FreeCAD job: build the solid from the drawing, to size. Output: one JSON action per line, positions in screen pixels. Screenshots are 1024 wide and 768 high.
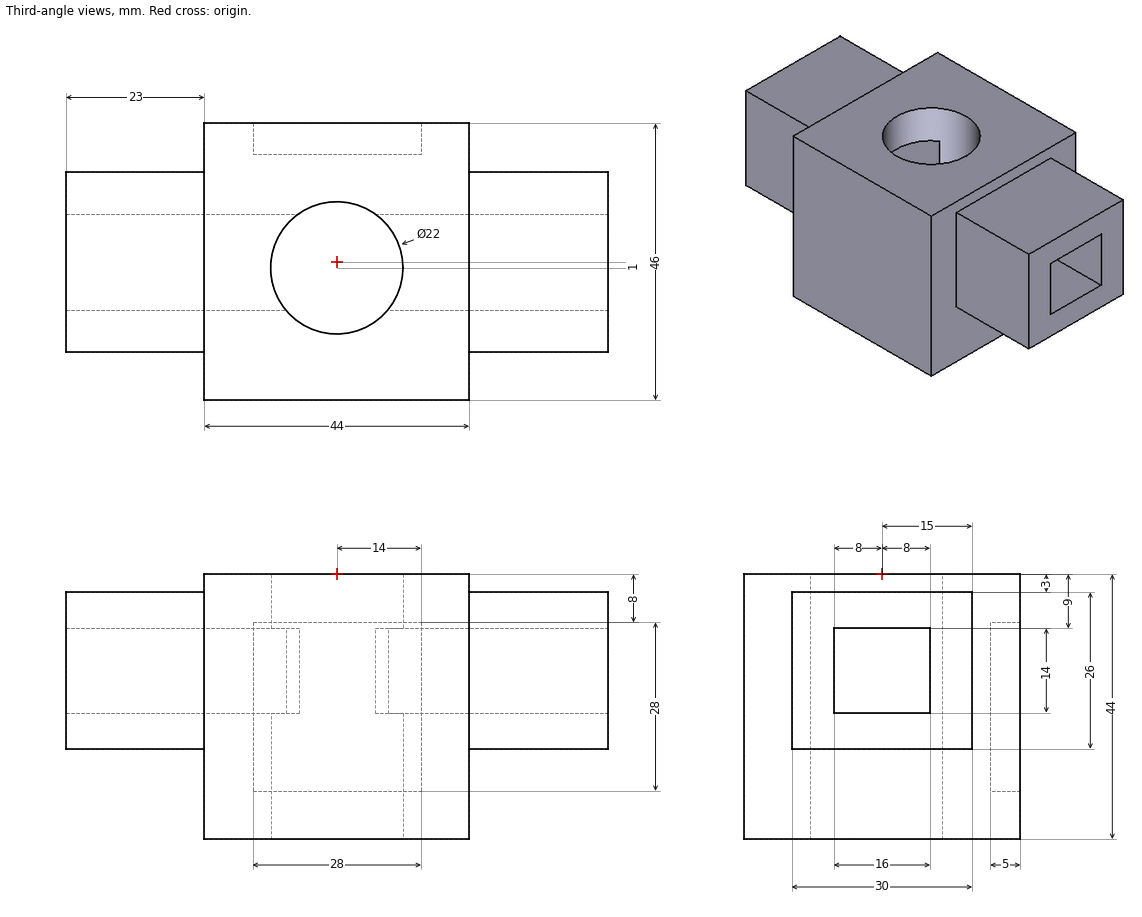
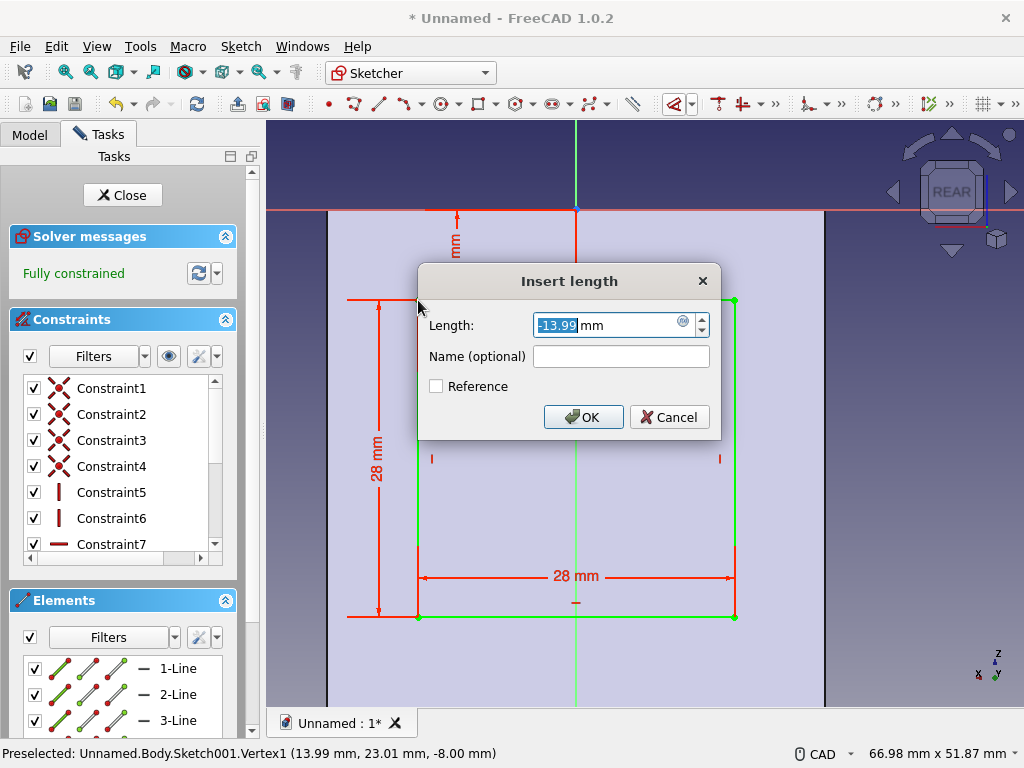
{"action": "type", "text": "-14"}
{"action": "key", "text": "Return"}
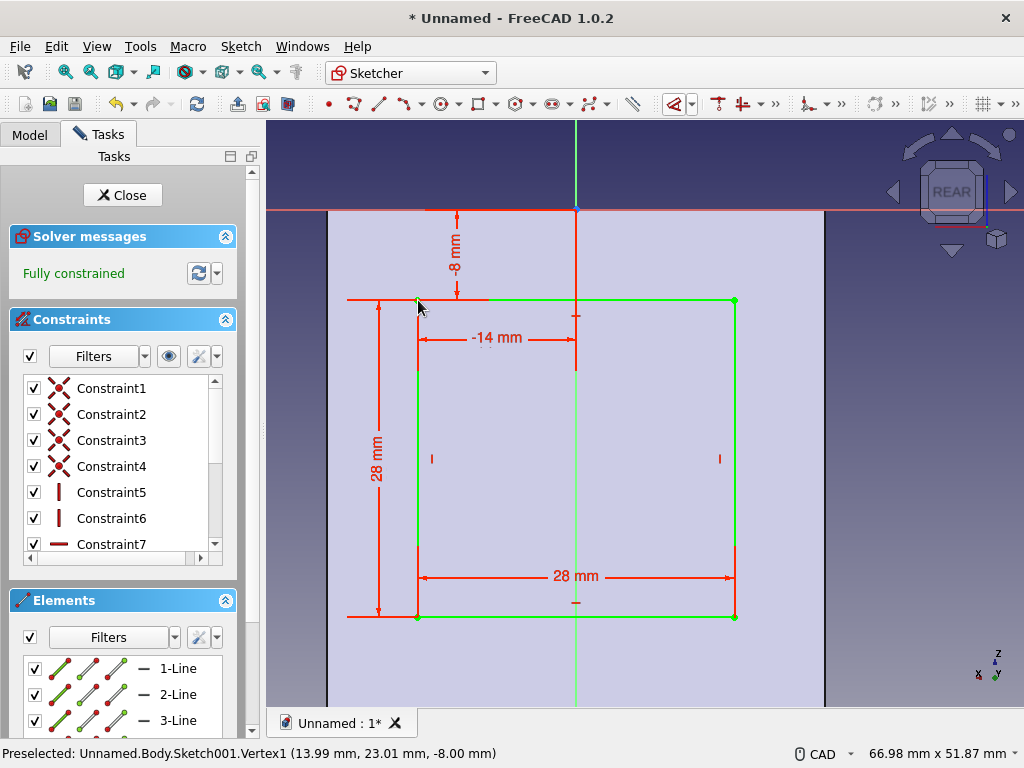
{"action": "left_click", "coordinate": [123, 195]}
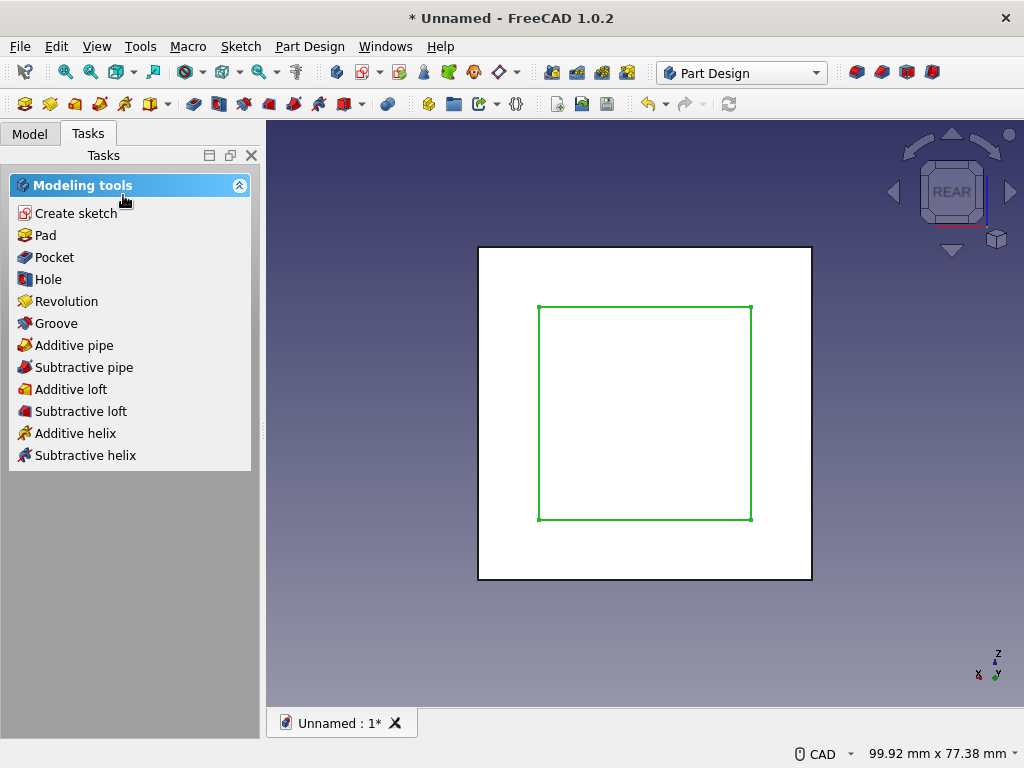
{"action": "left_click", "coordinate": [194, 104]}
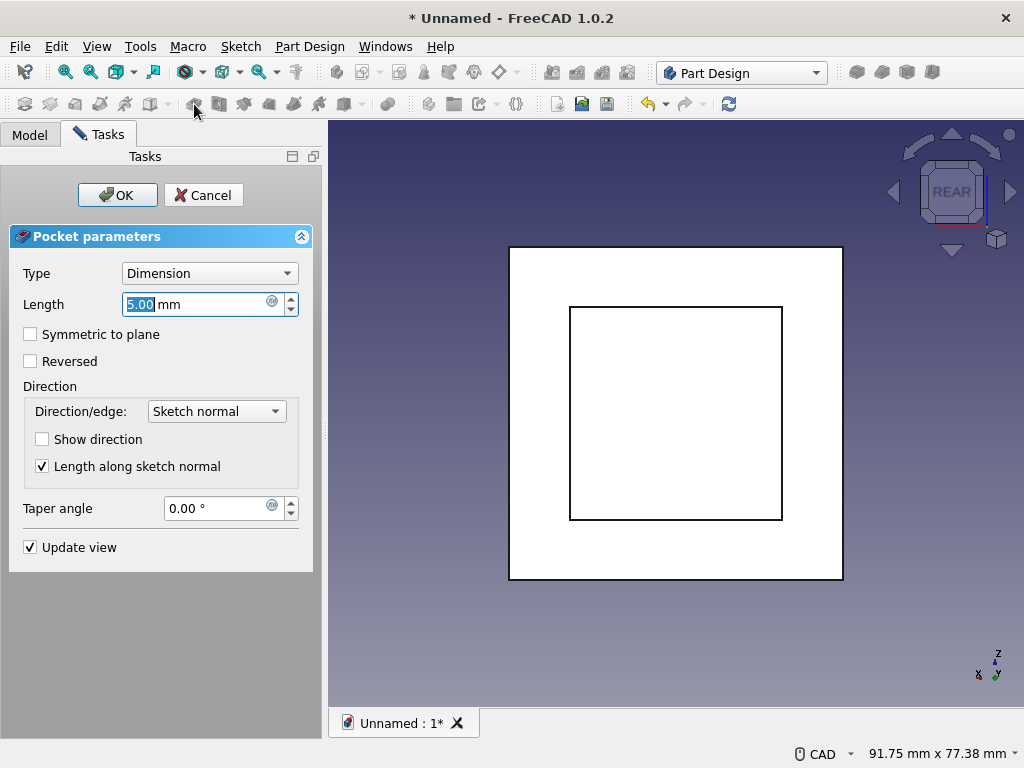
{"action": "type", "text": "5"}
{"action": "key", "text": "Tab"}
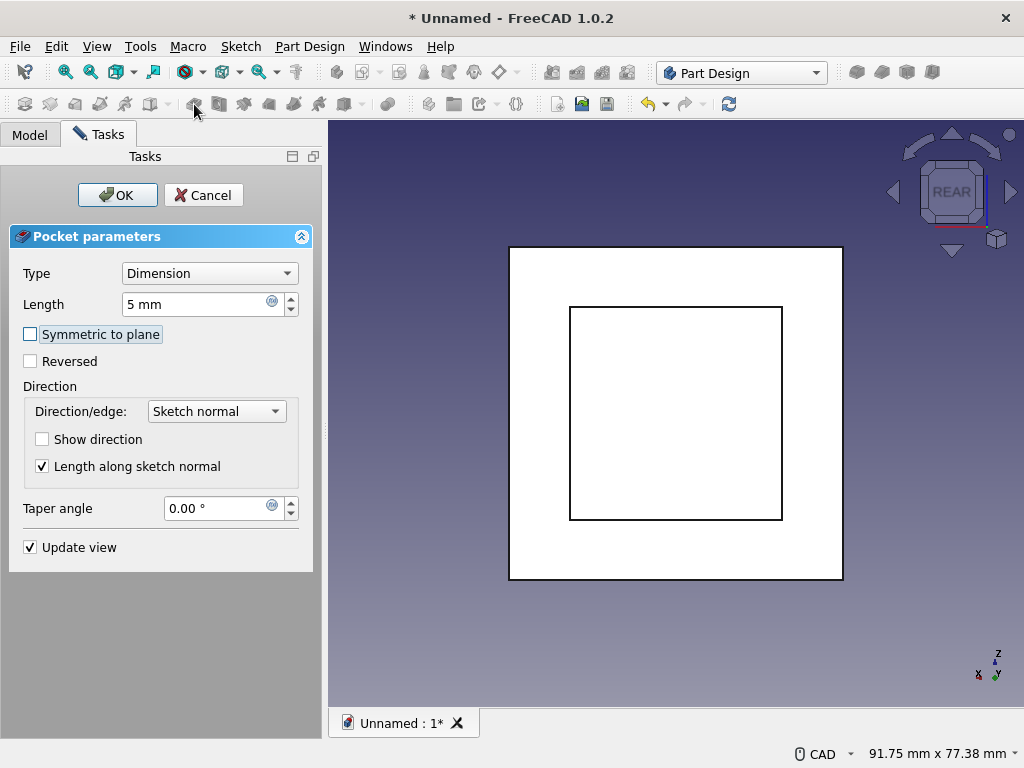
{"action": "left_click", "coordinate": [118, 195]}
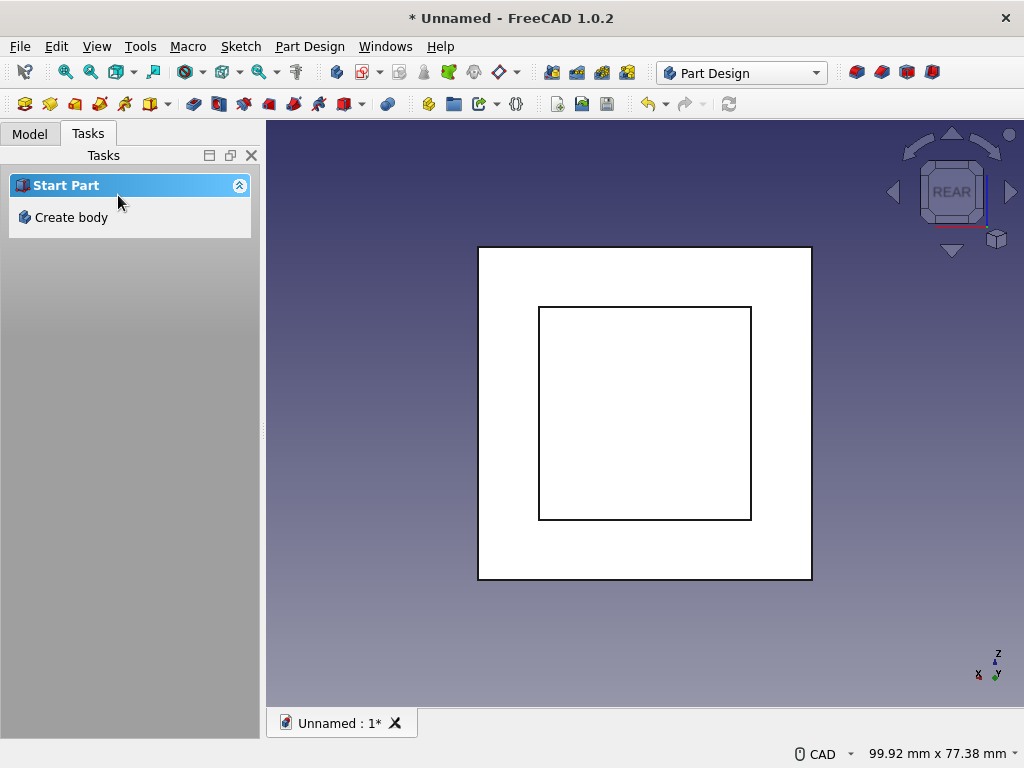
{"action": "key", "text": "6"}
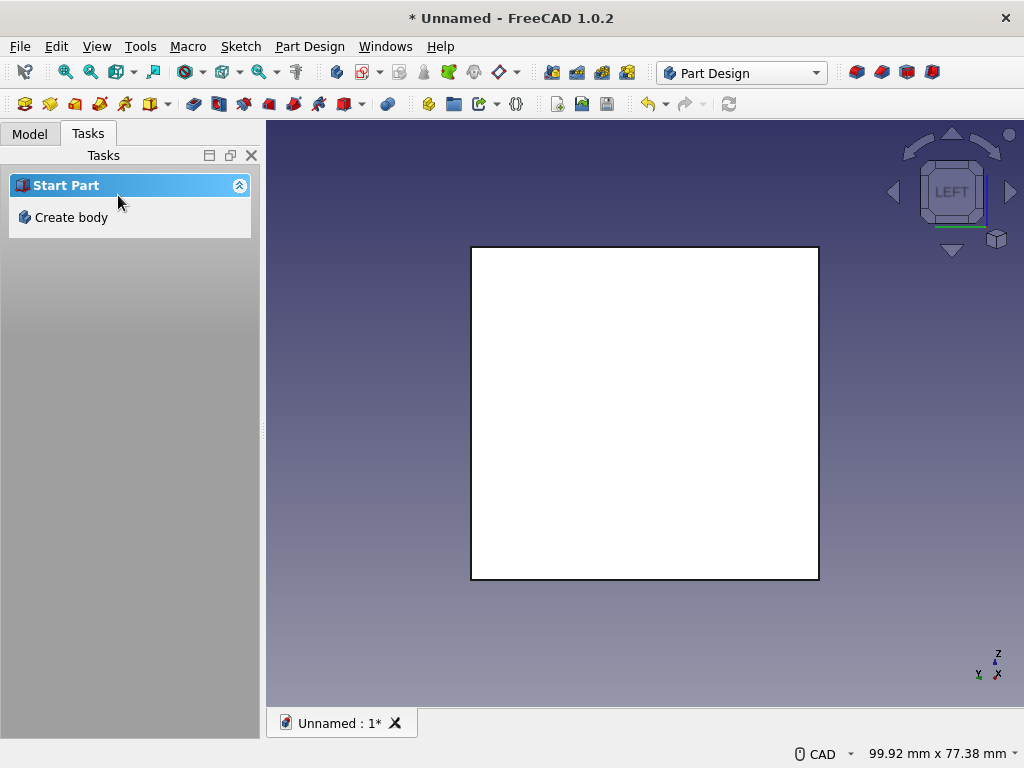
{"action": "left_click", "coordinate": [645, 413]}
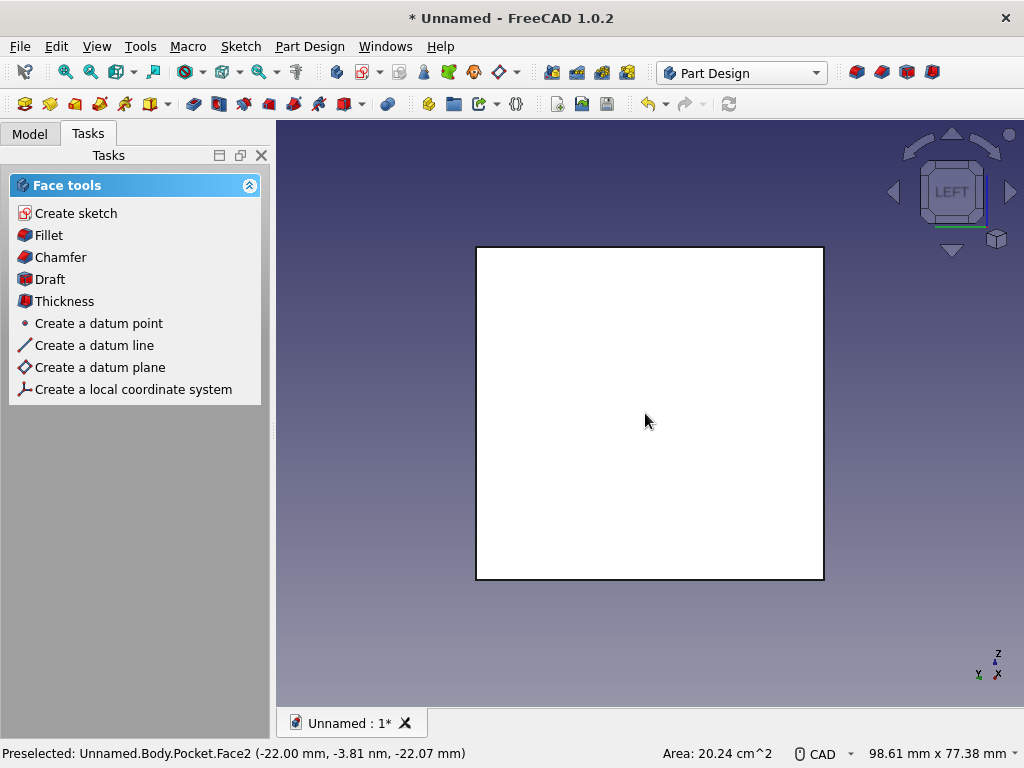
{"action": "left_click", "coordinate": [362, 72]}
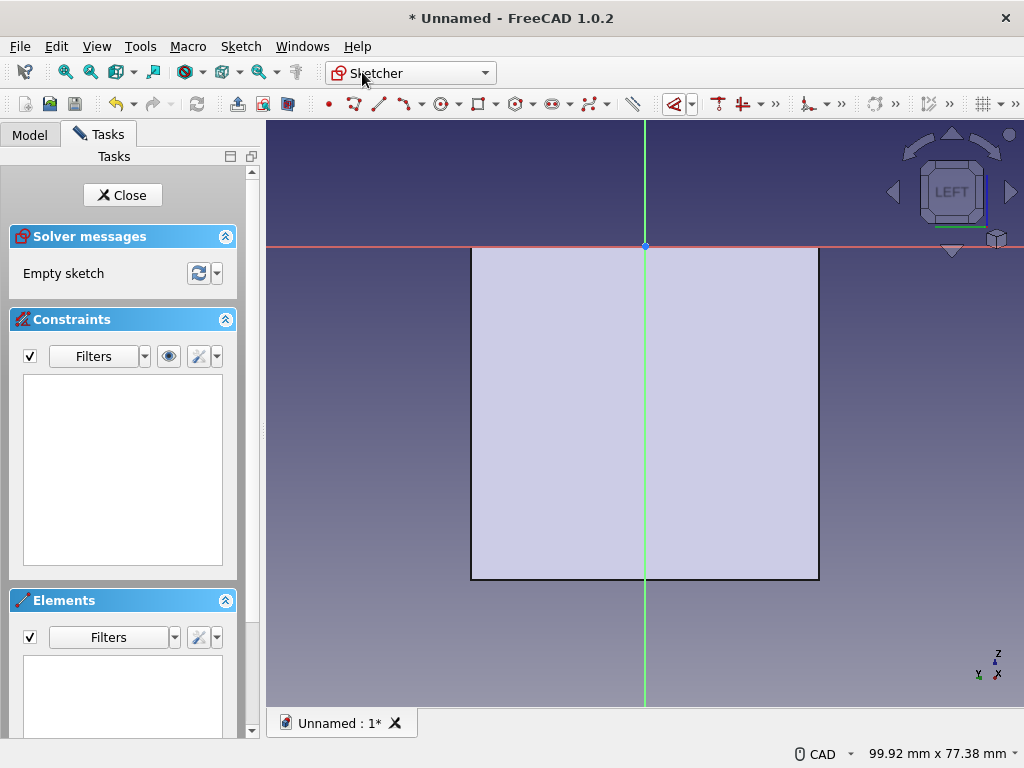
{"action": "scroll", "coordinate": [728, 287], "scroll_direction": "up", "scroll_amount": 3}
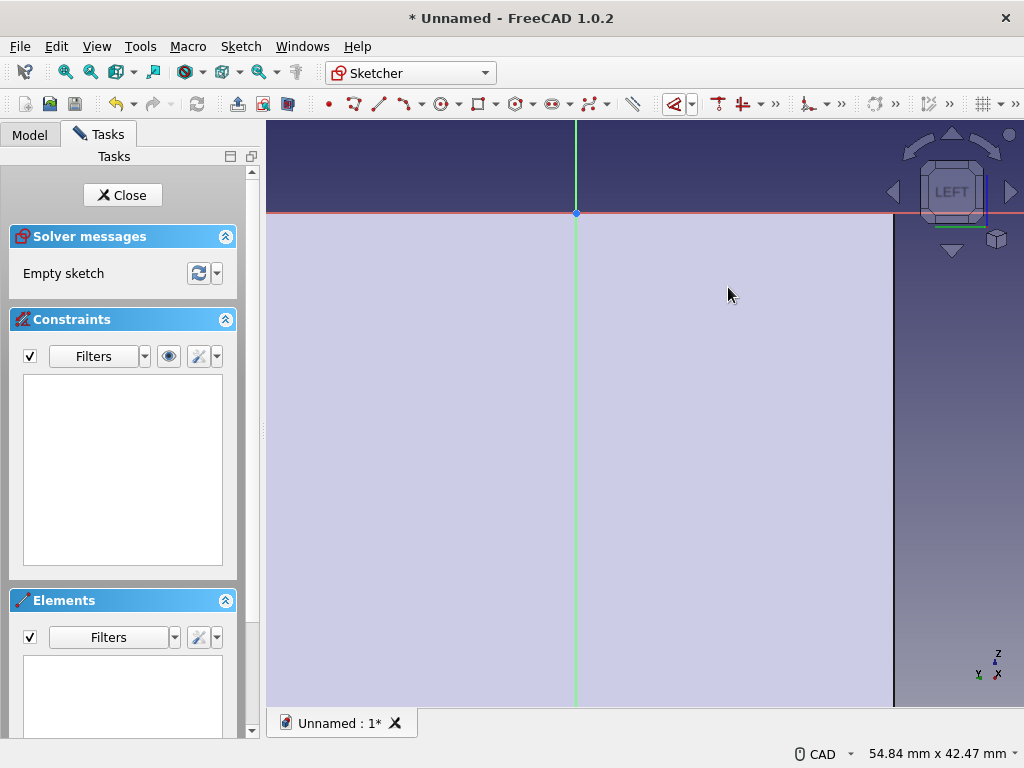
{"action": "key", "text": "g r"}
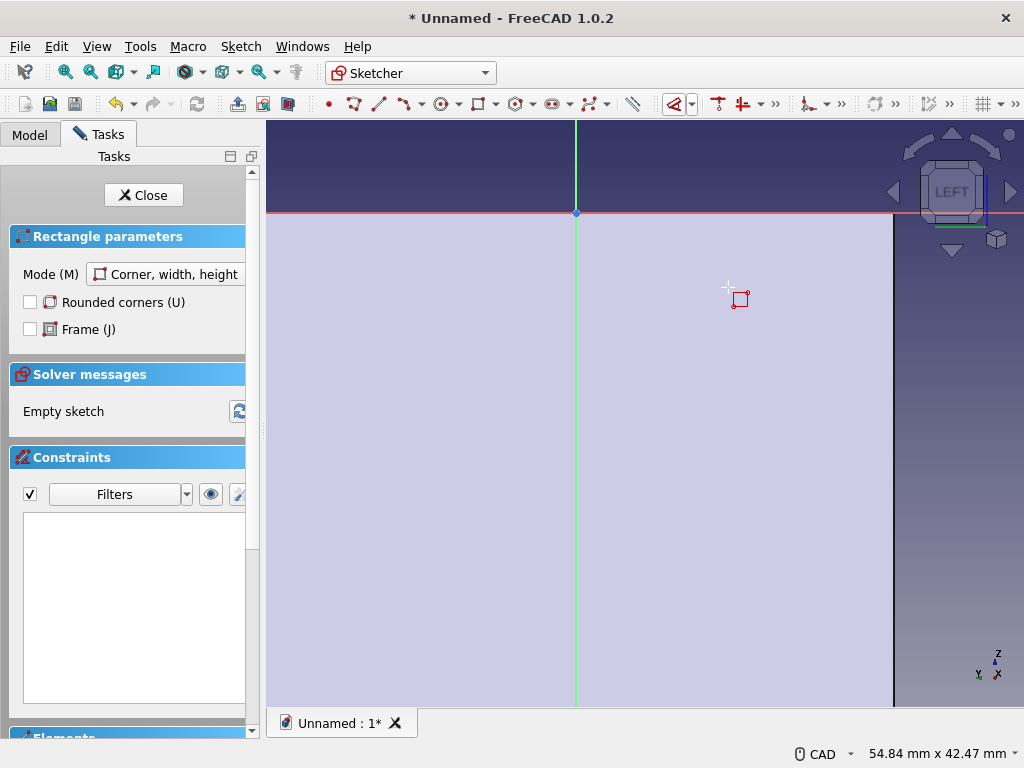
{"action": "left_click", "coordinate": [369, 255]}
{"action": "left_click", "coordinate": [784, 614]}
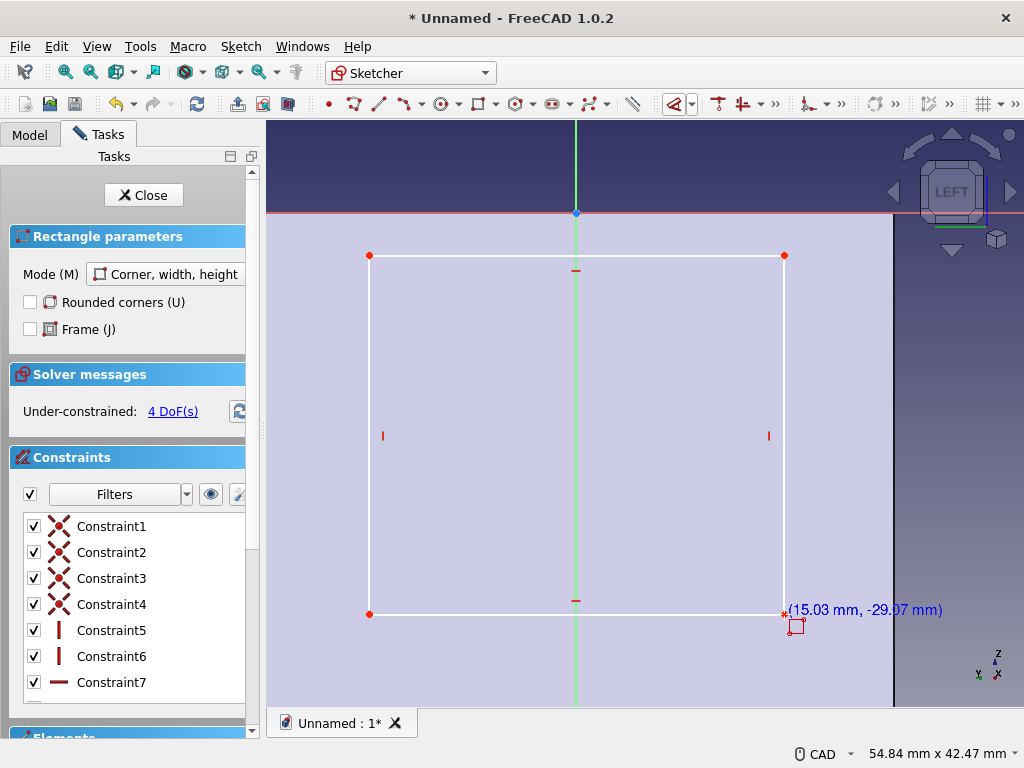
{"action": "left_click", "coordinate": [466, 338]}
{"action": "left_click", "coordinate": [687, 531]}
{"action": "key", "text": "Escape"}